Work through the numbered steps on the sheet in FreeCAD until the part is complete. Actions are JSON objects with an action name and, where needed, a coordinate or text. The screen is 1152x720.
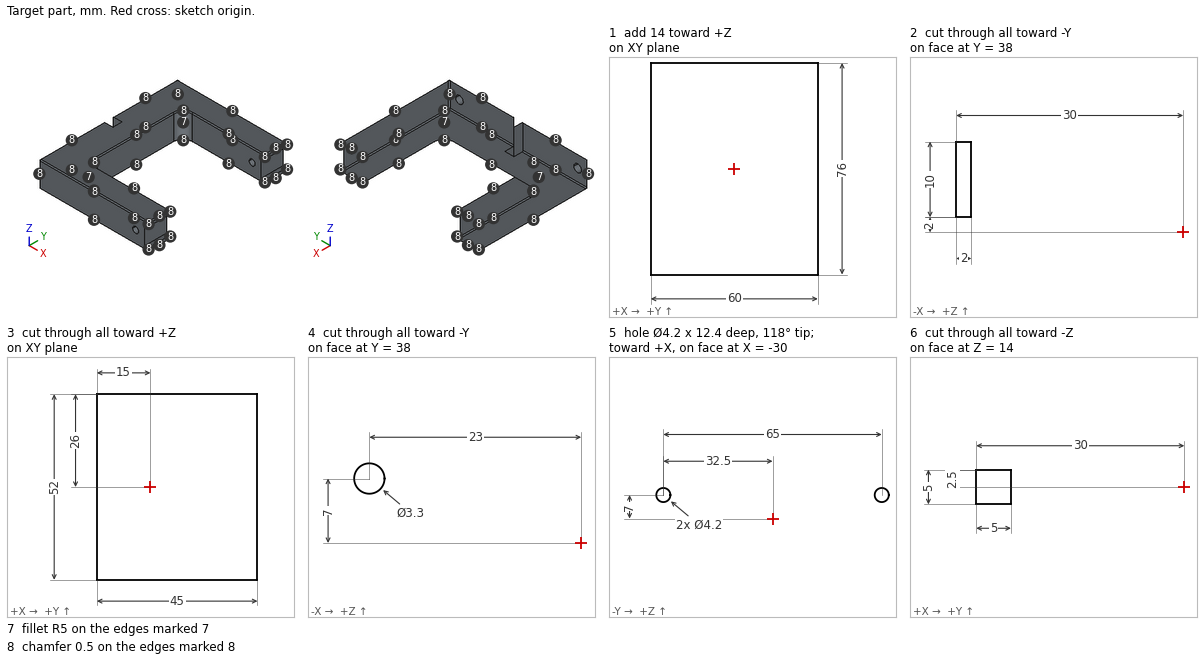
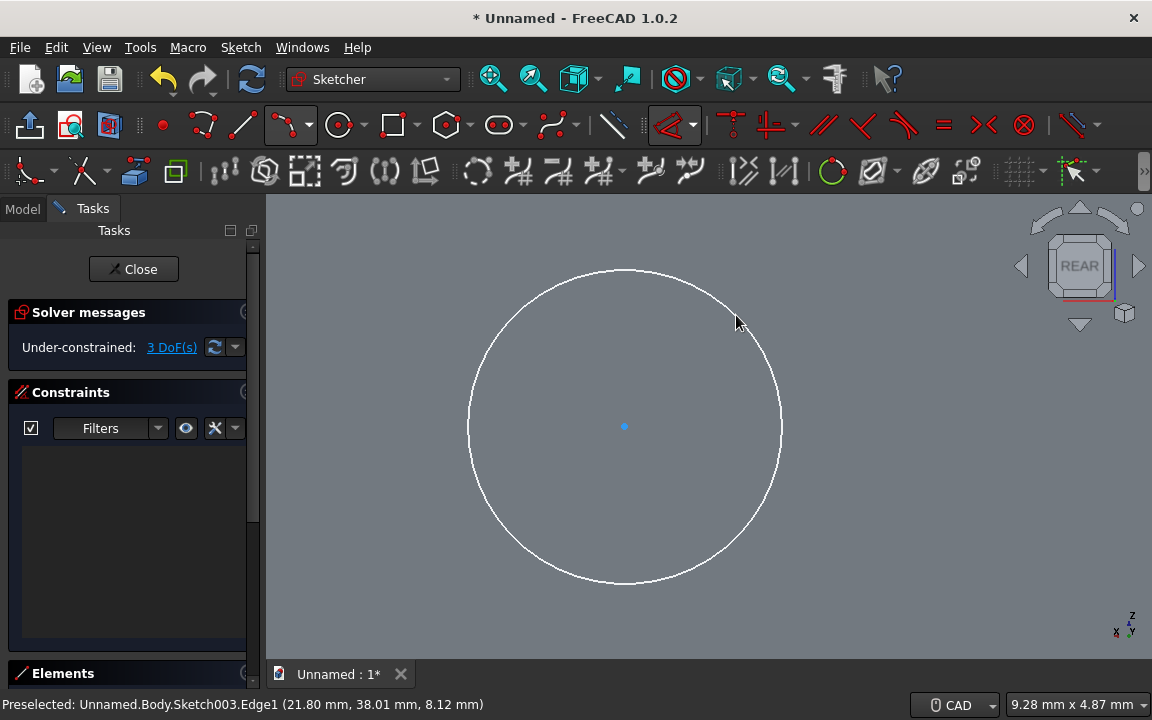
{"action": "left_click", "coordinate": [736, 316]}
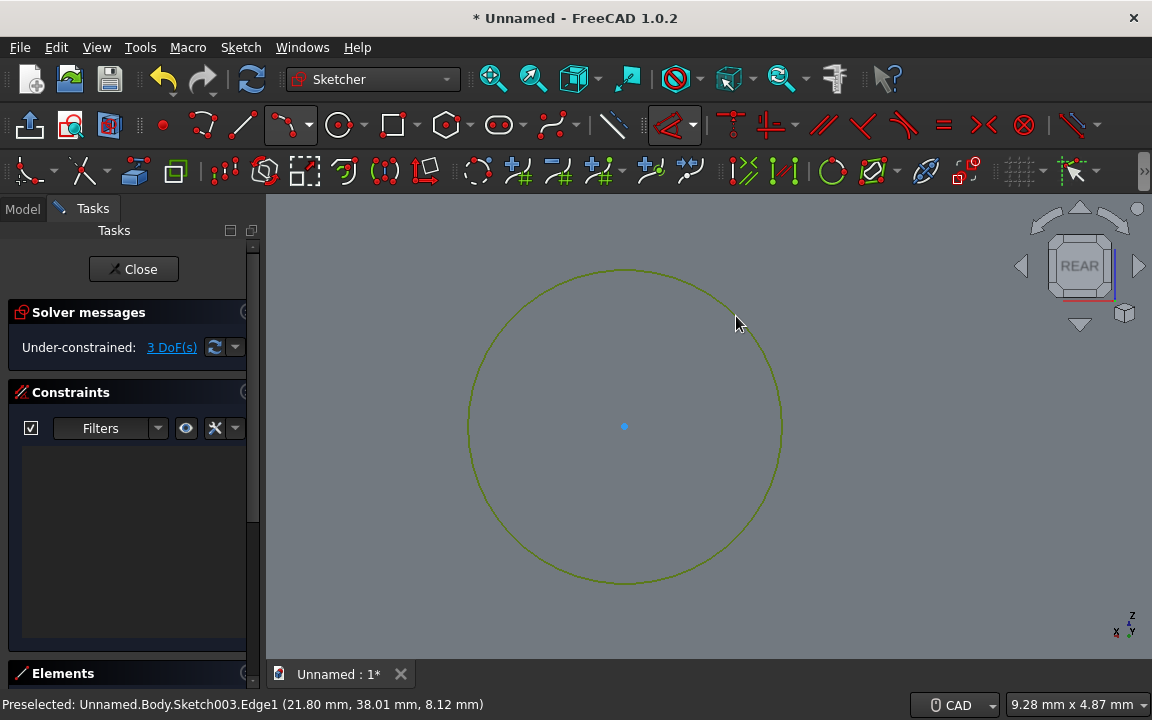
{"action": "key", "text": "k o"}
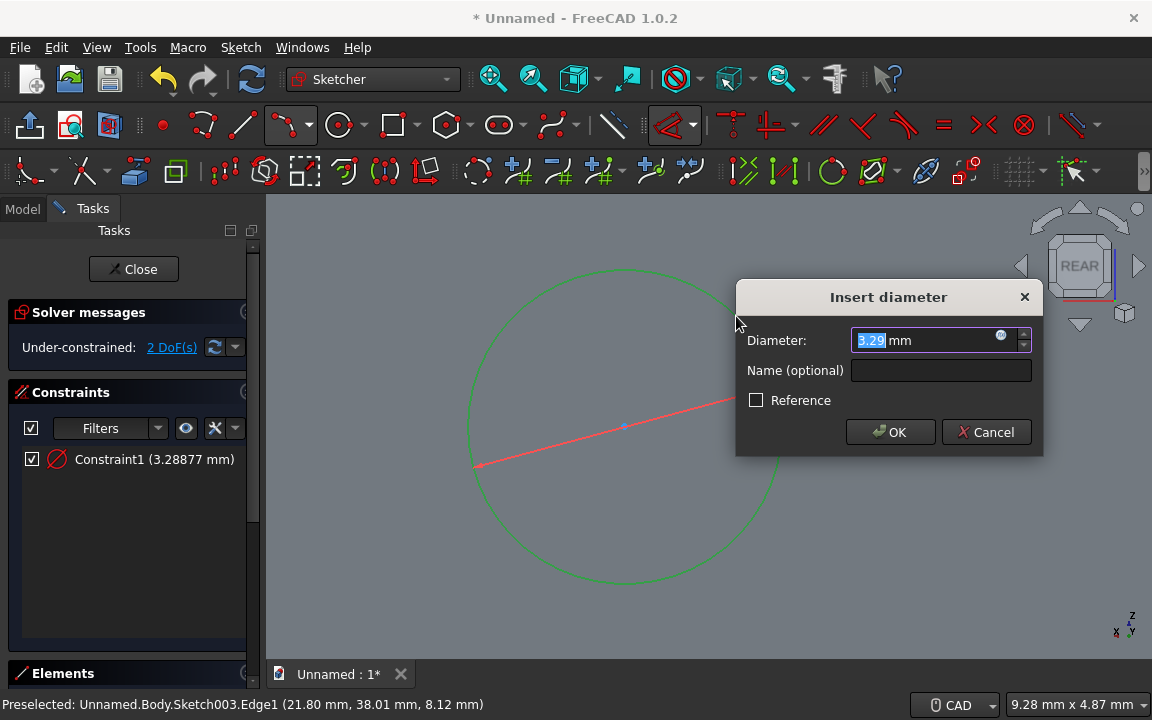
{"action": "type", "text": "3.3"}
{"action": "key", "text": "Return"}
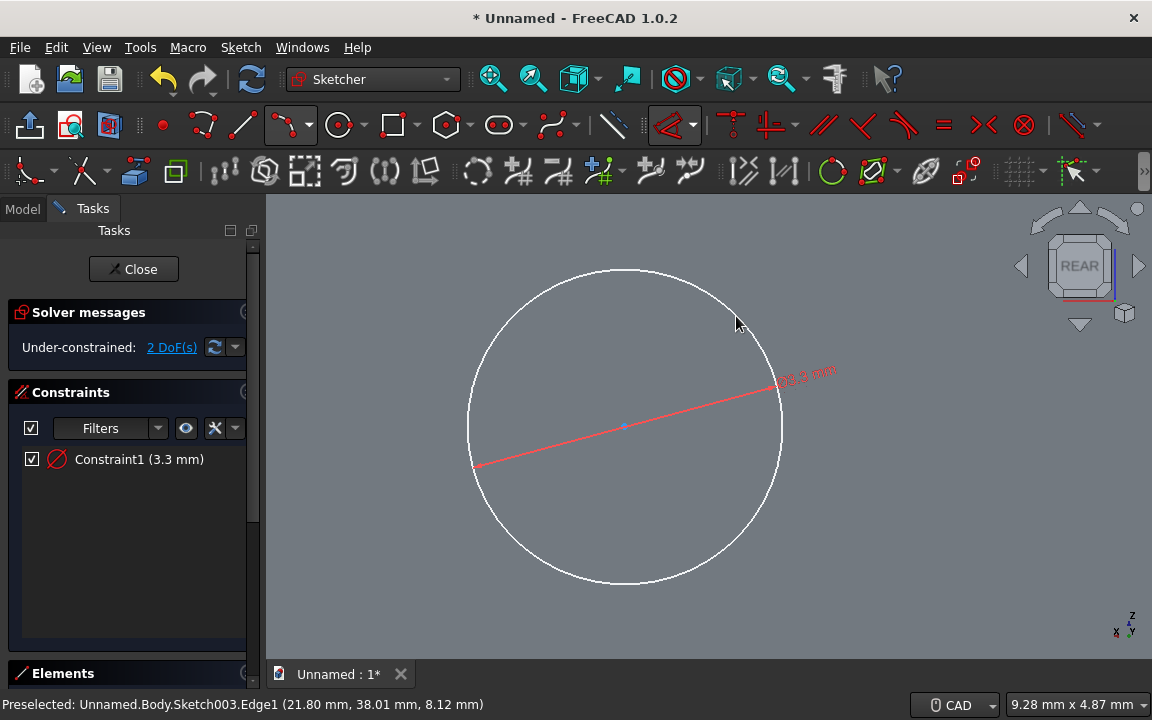
{"action": "left_click", "coordinate": [625, 427]}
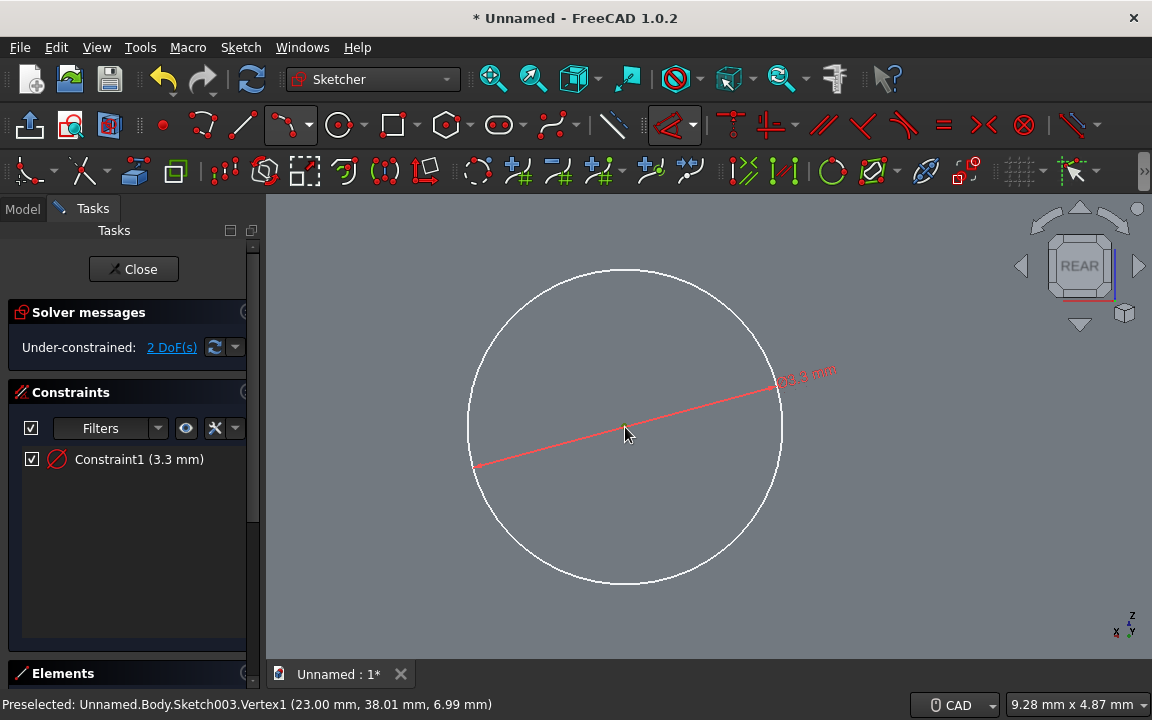
{"action": "key", "text": "i"}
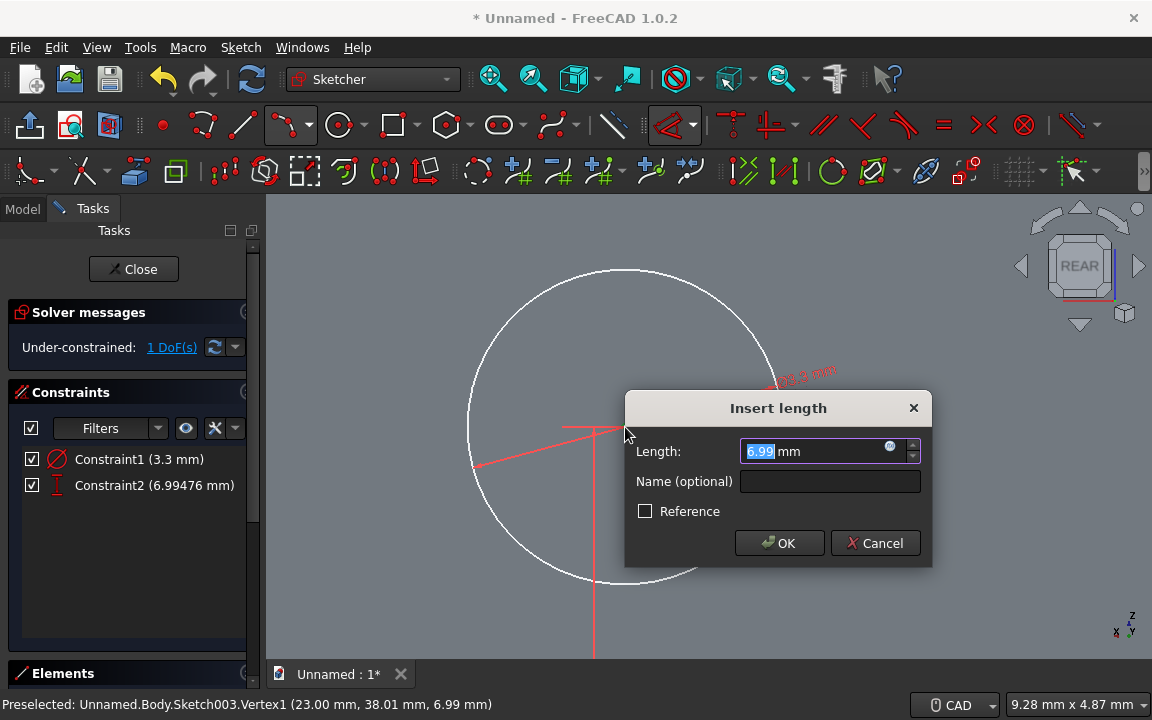
{"action": "type", "text": "7"}
{"action": "key", "text": "Return"}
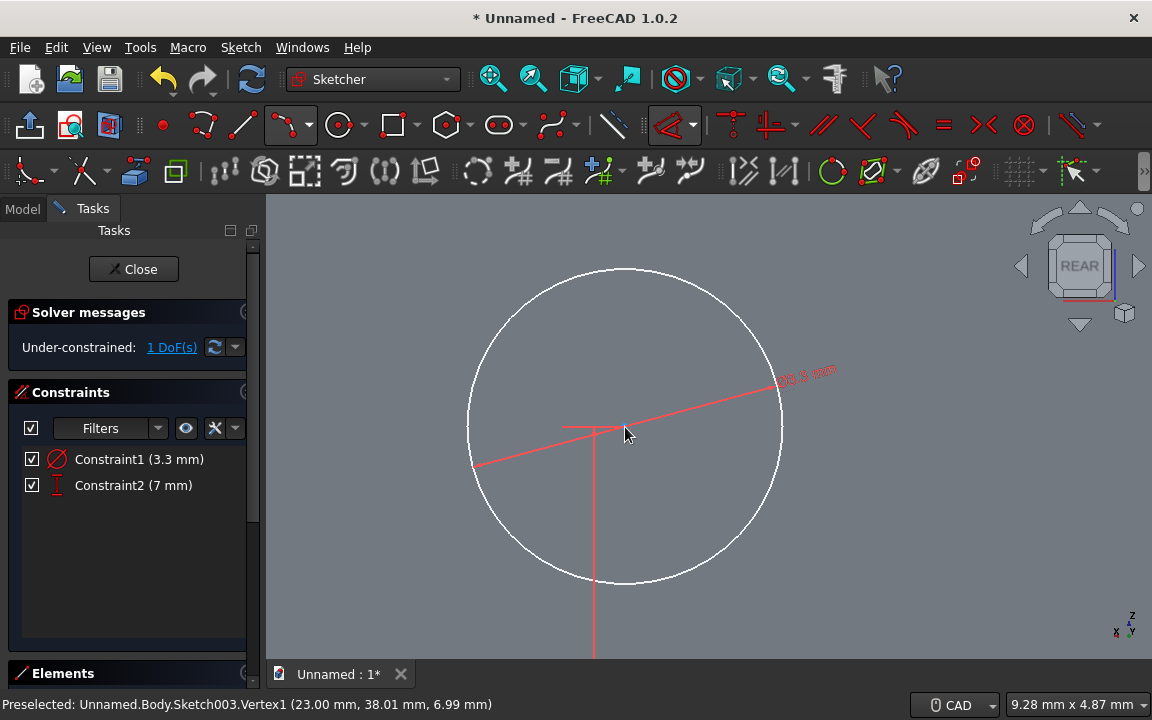
{"action": "left_click", "coordinate": [625, 426]}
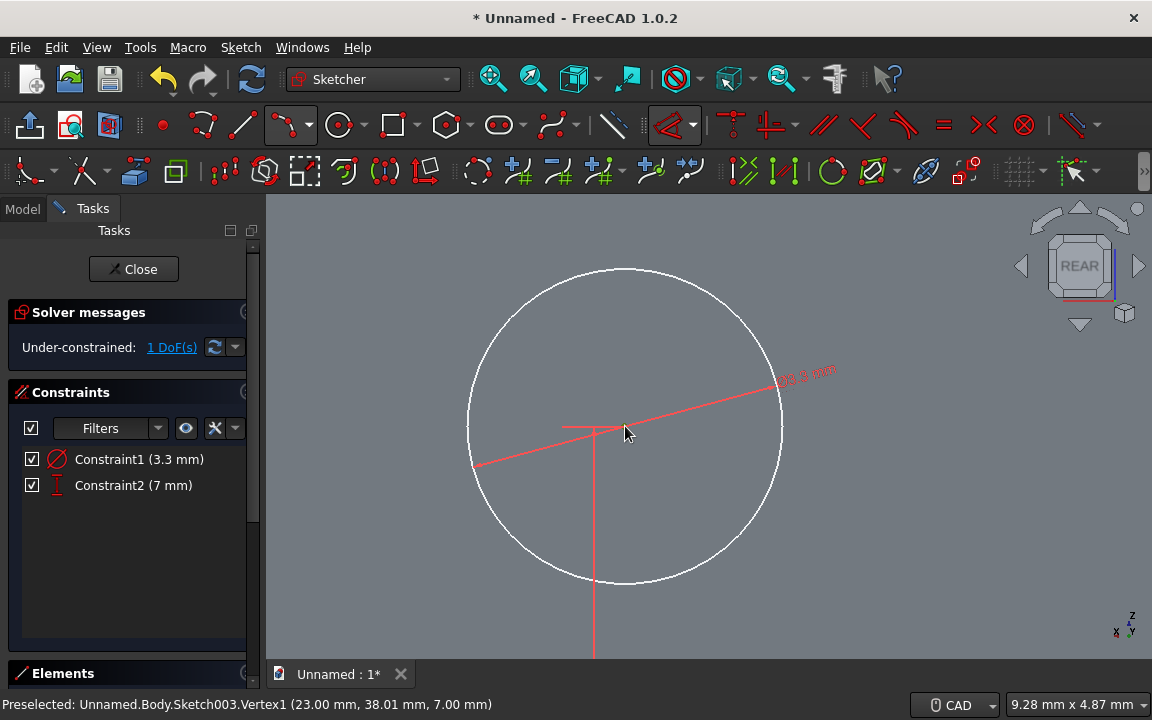
{"action": "key", "text": "l"}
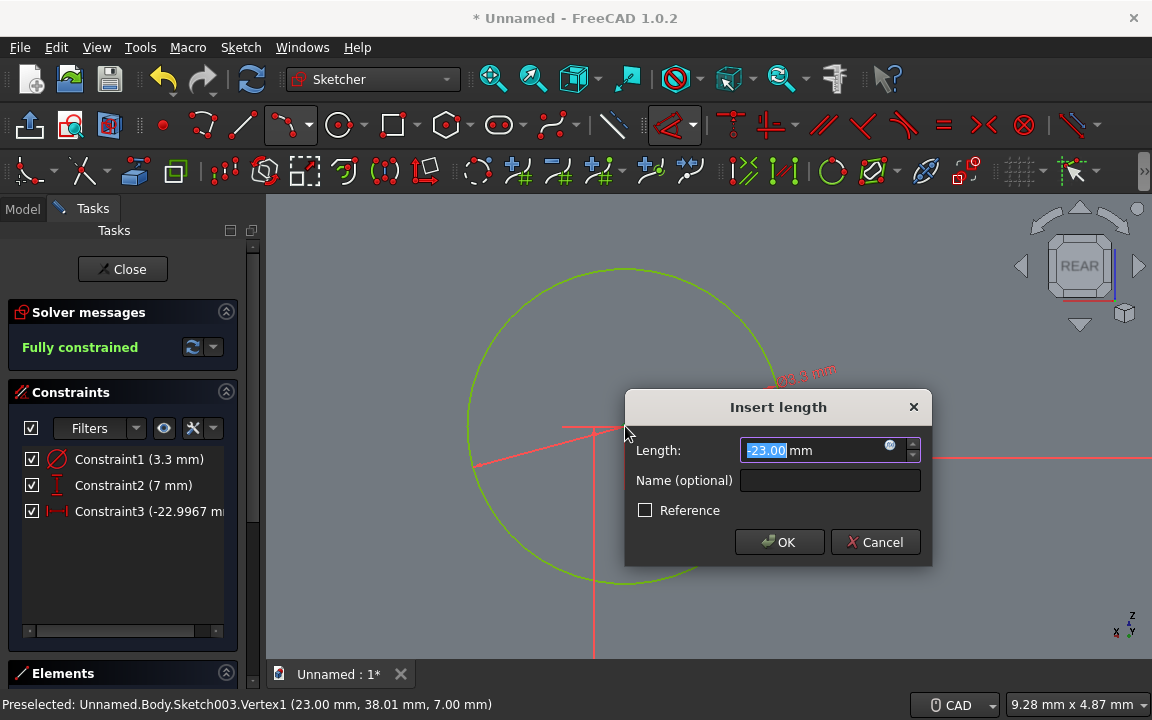
{"action": "type", "text": "-23"}
{"action": "key", "text": "Return"}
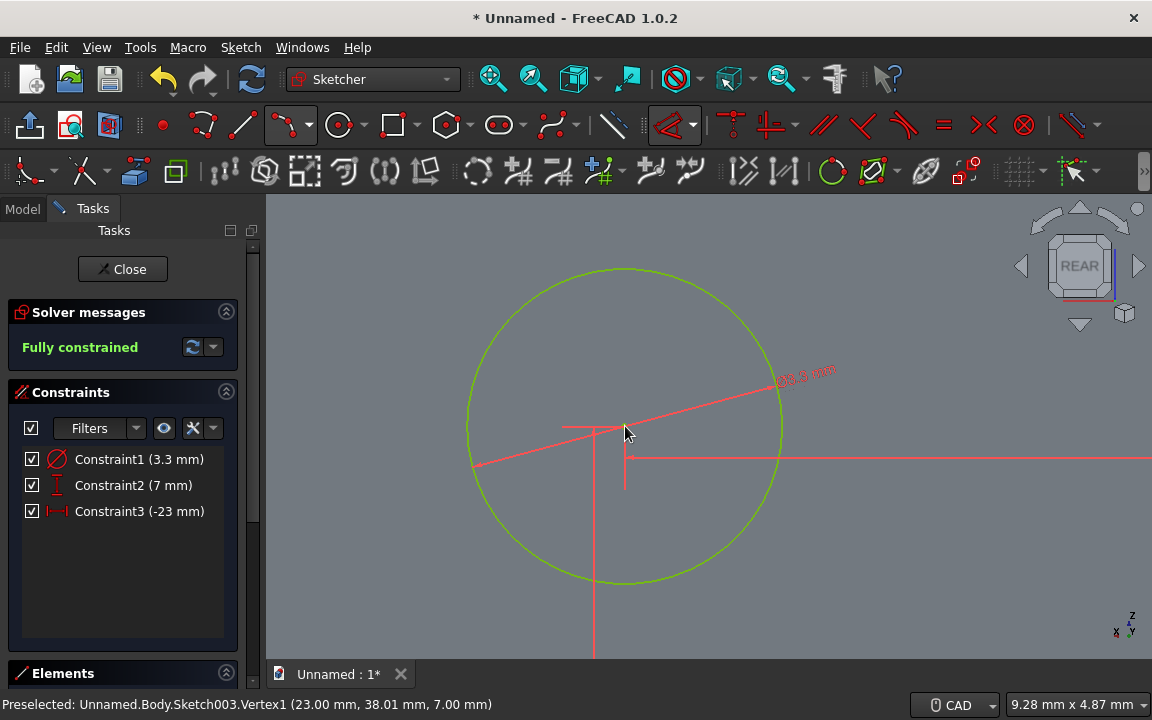
{"action": "left_click", "coordinate": [123, 269]}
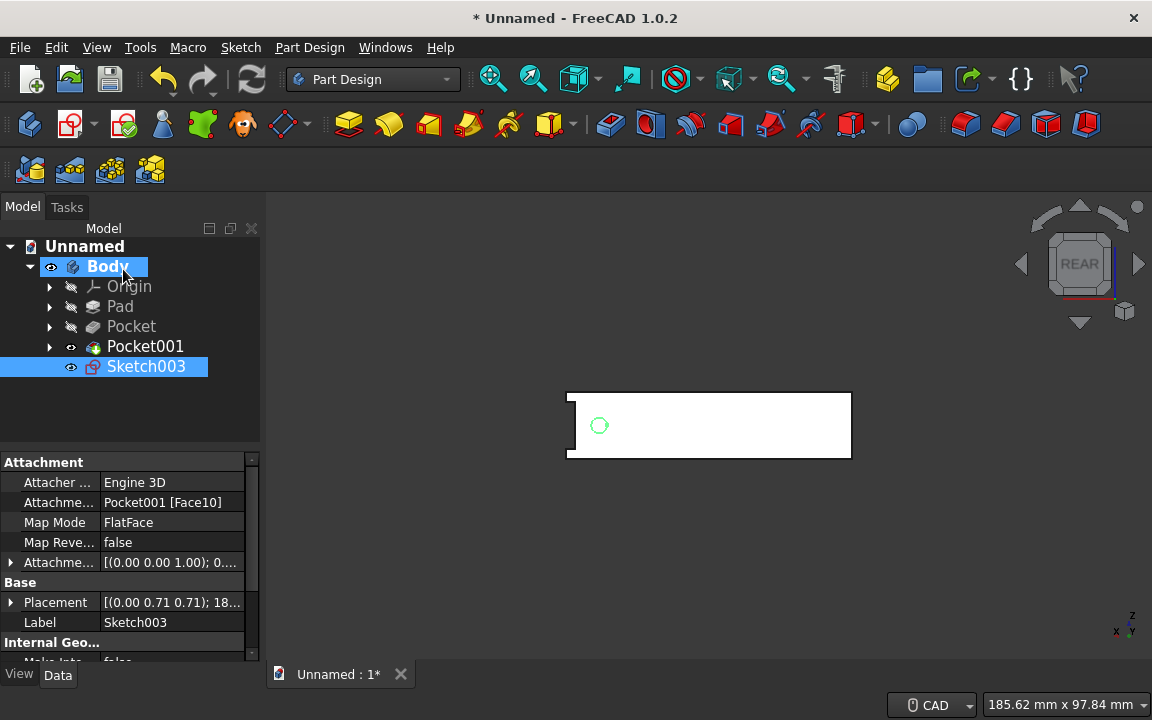
{"action": "left_click", "coordinate": [612, 124]}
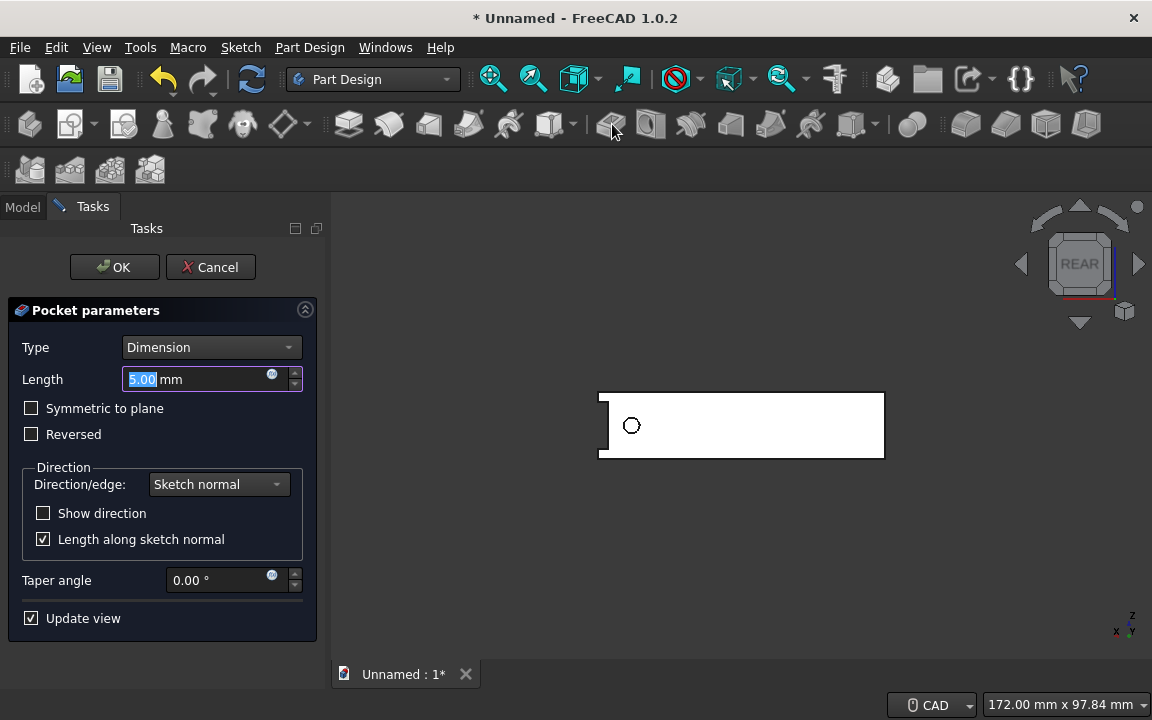
{"action": "left_click", "coordinate": [212, 348]}